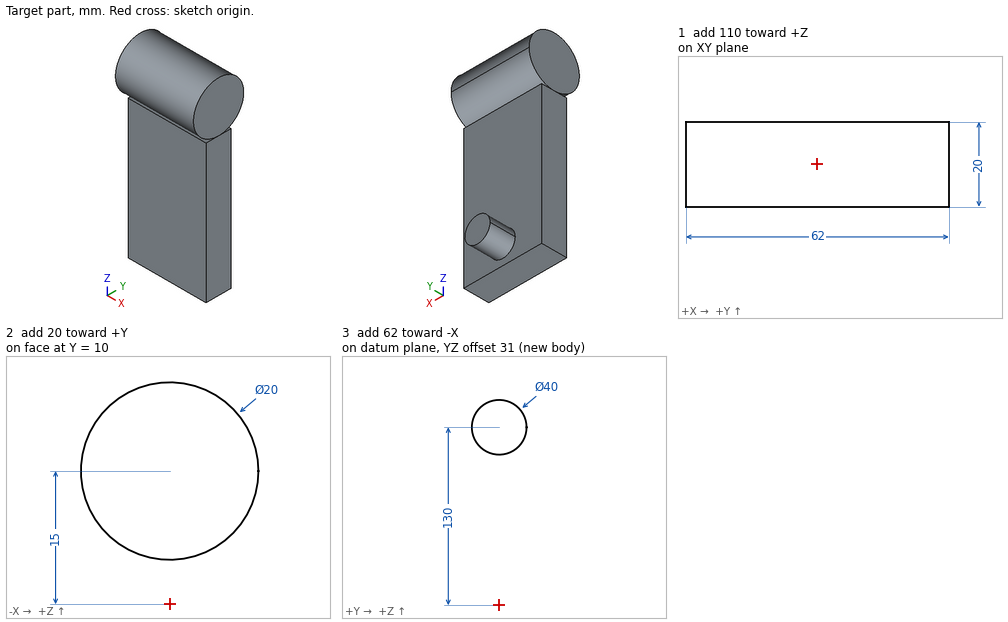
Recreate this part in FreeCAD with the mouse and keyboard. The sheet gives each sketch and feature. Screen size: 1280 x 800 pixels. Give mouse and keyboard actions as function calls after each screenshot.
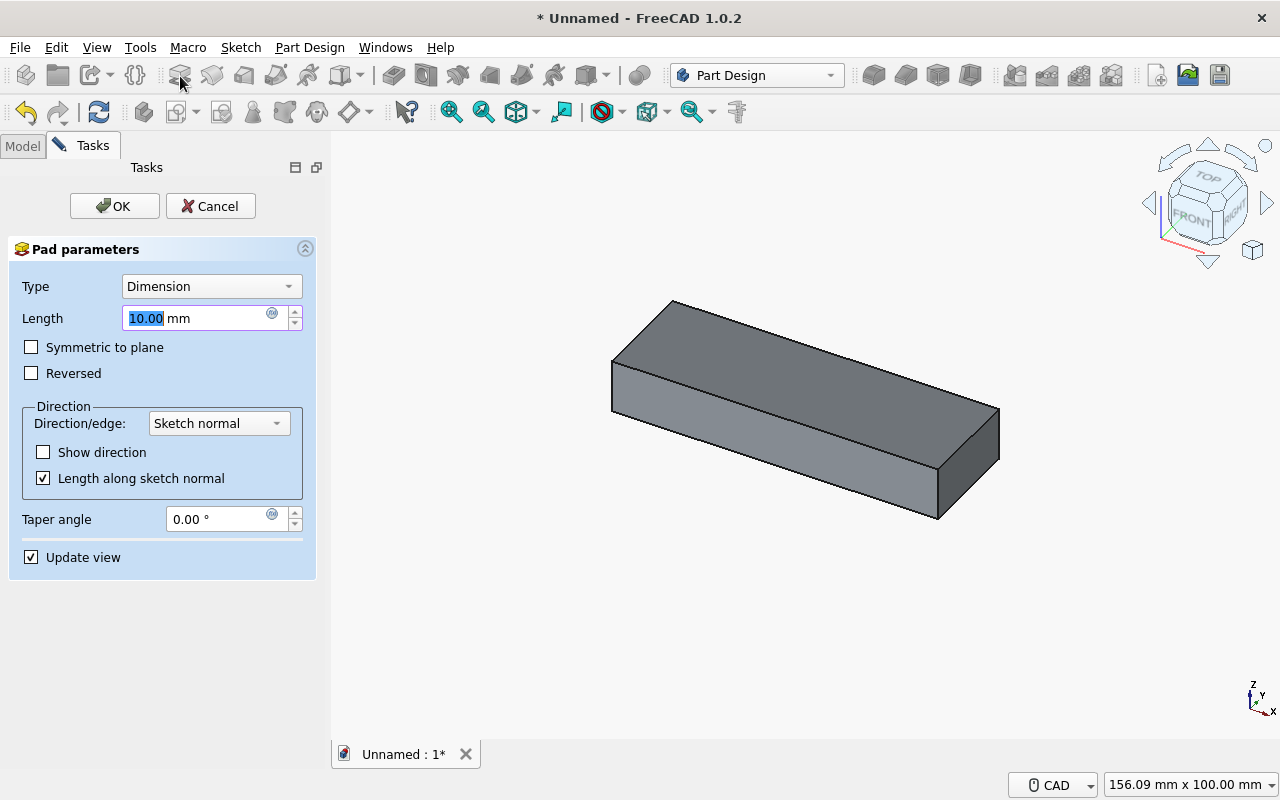
text(110)
key(Tab)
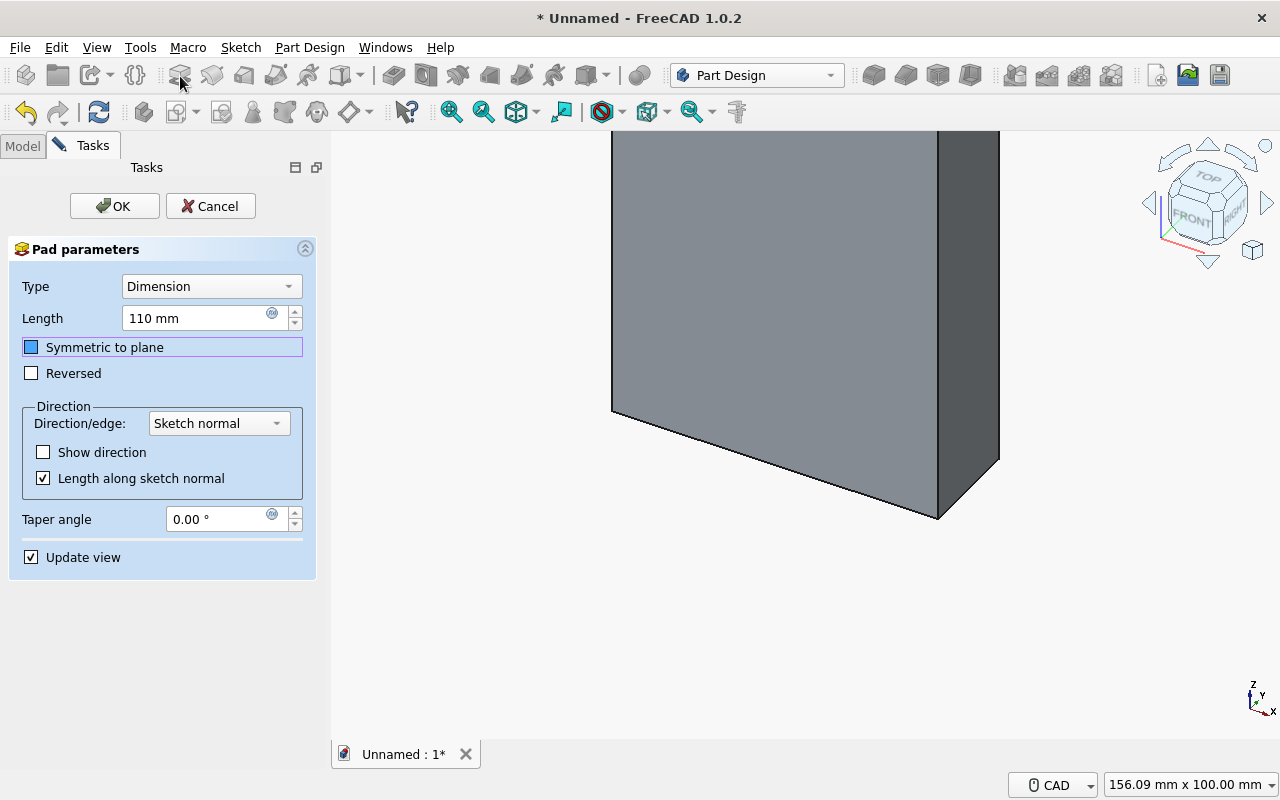
click(115, 206)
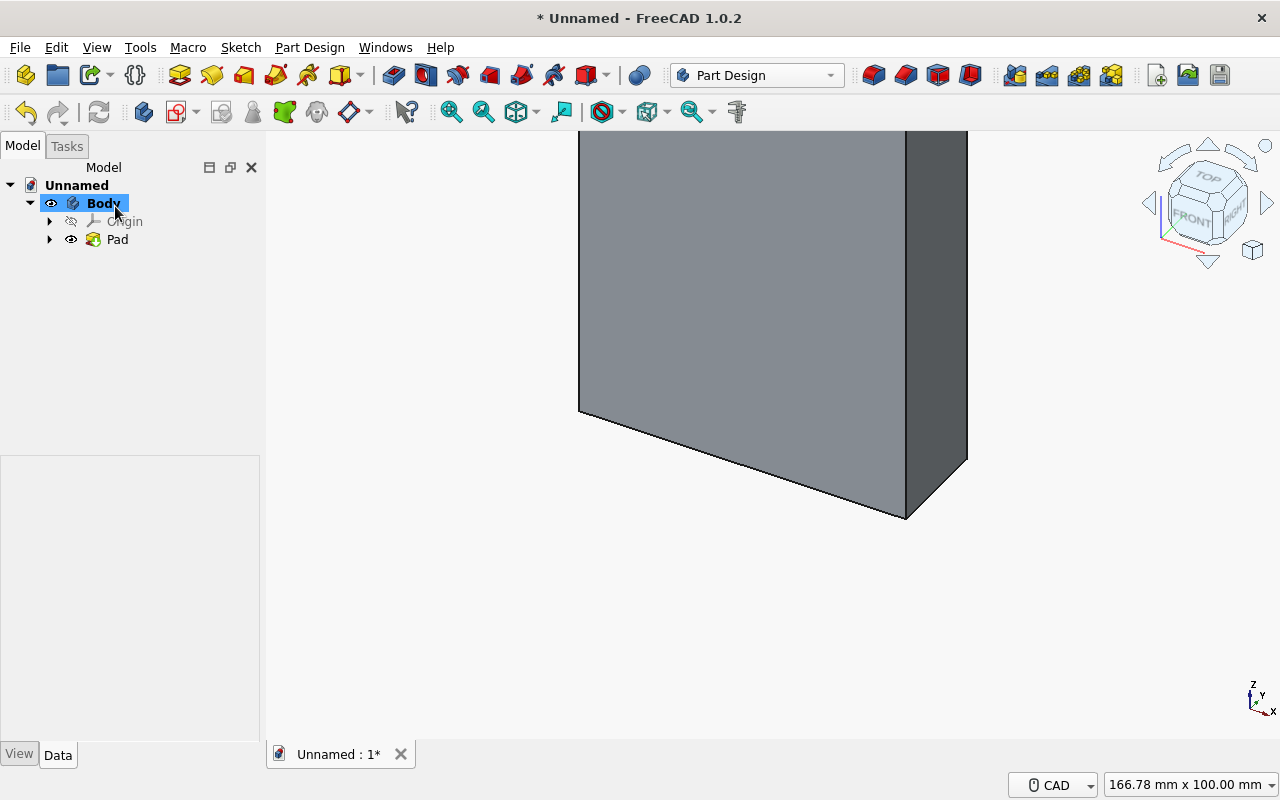
click(452, 112)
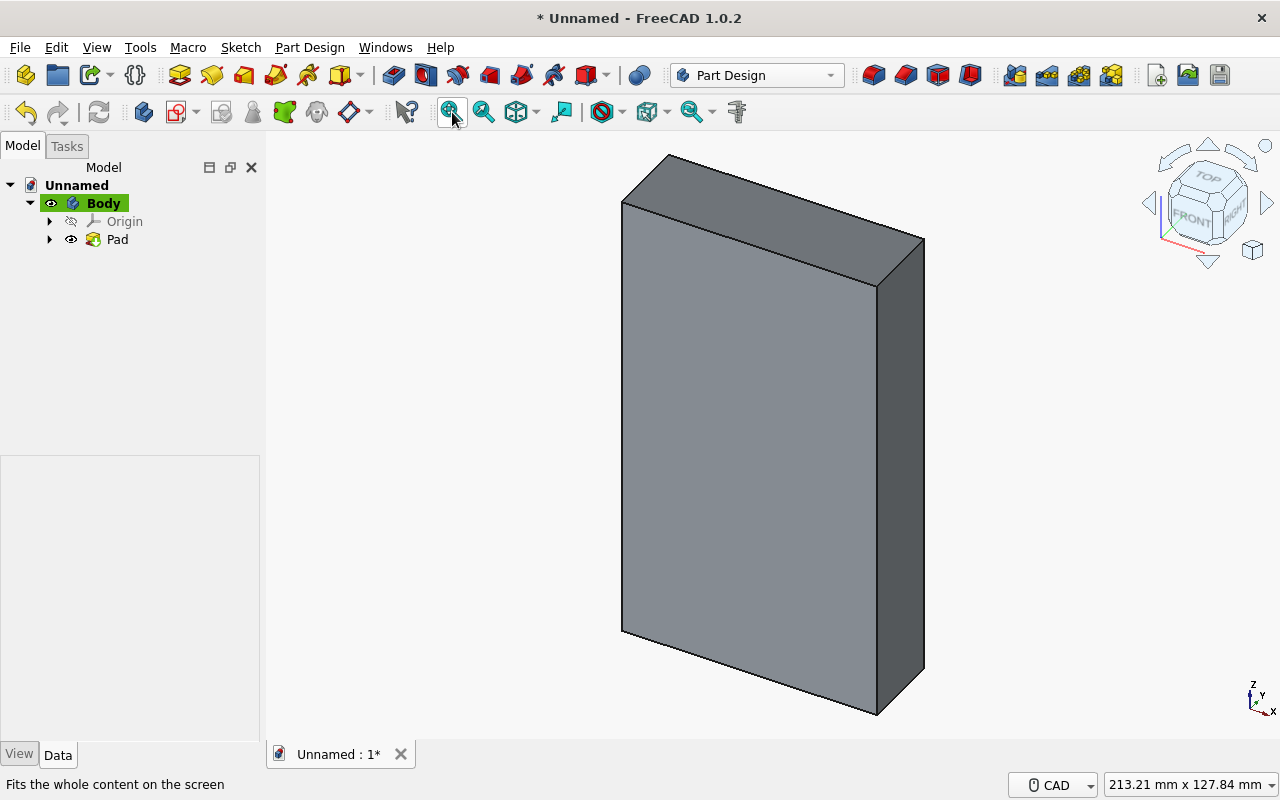
key(4)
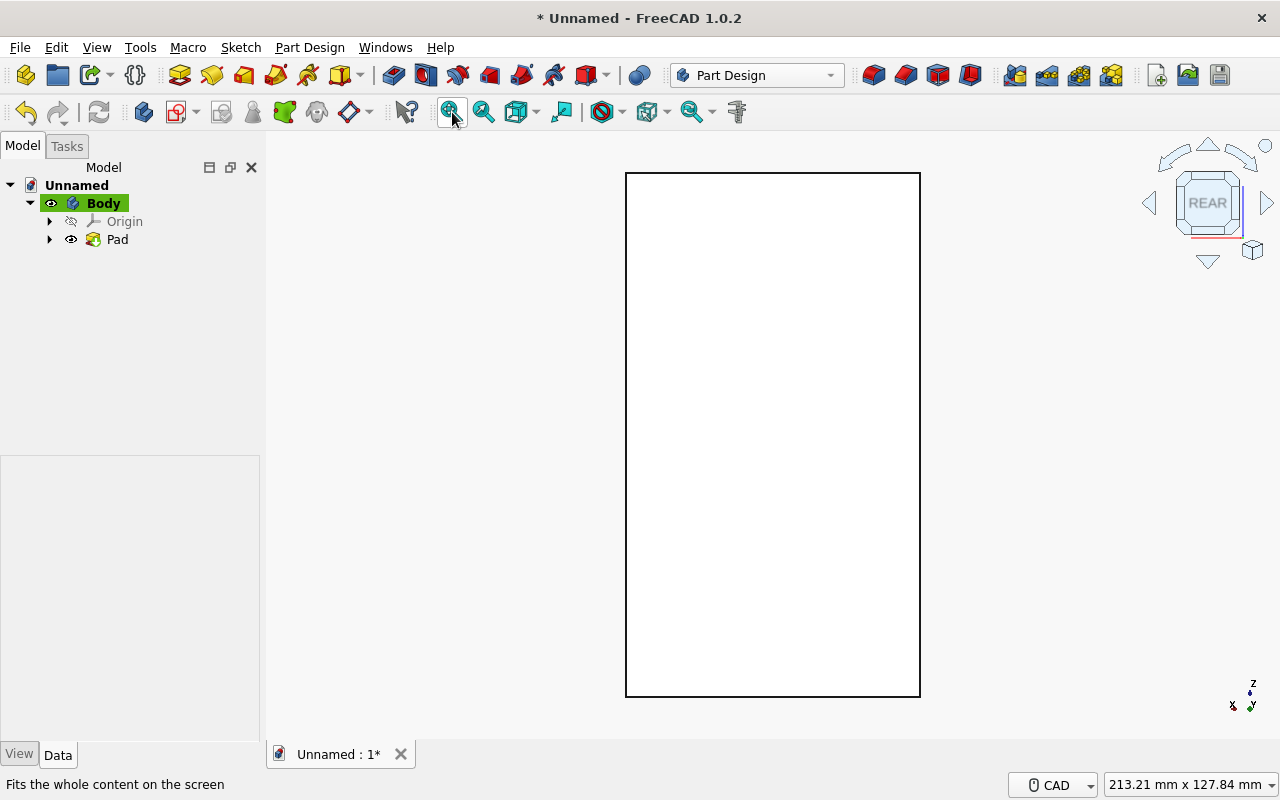
click(773, 359)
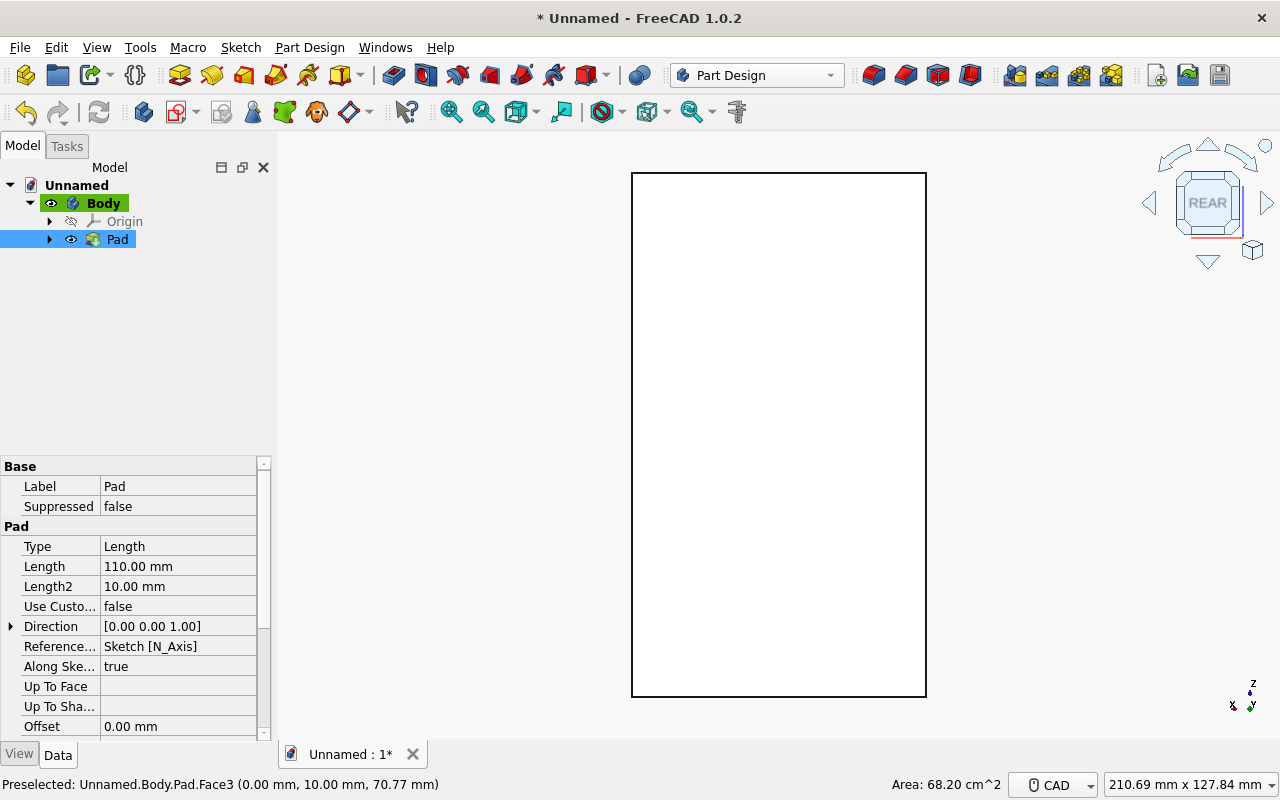
click(176, 112)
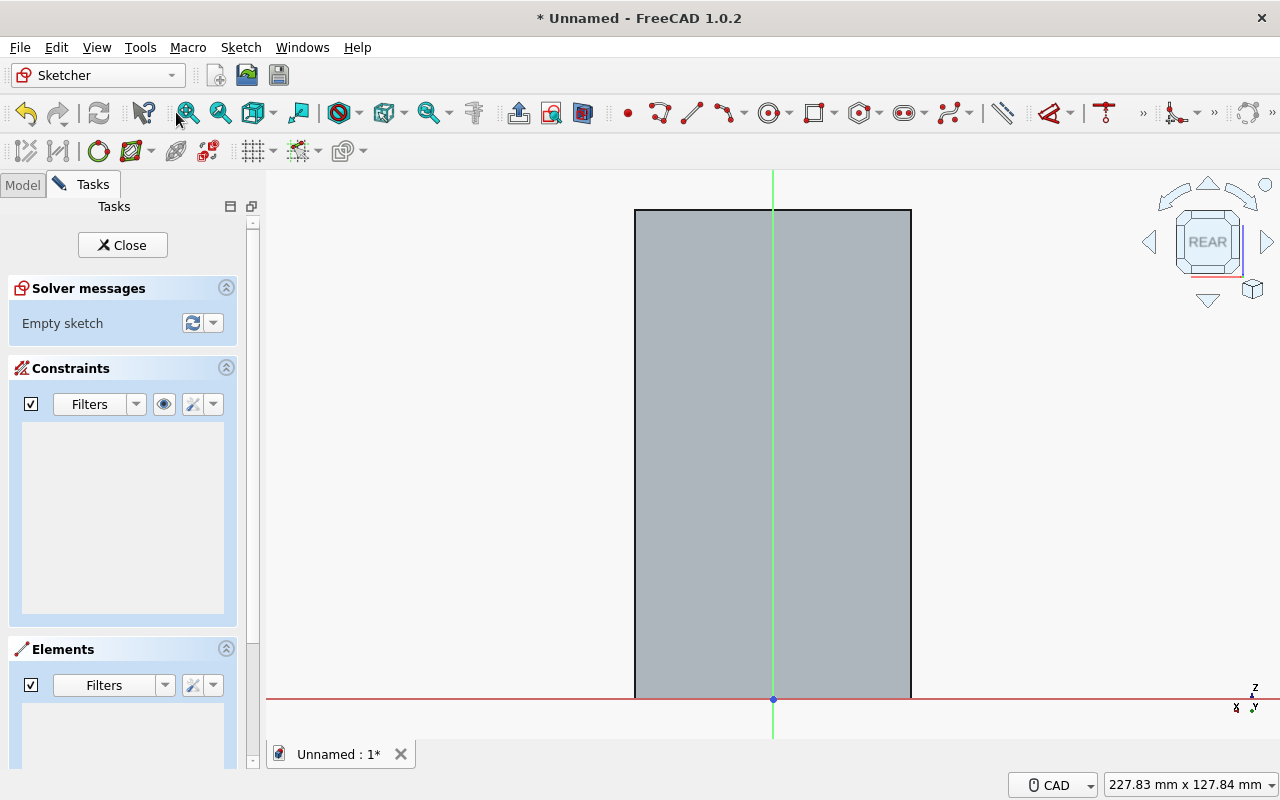
scroll(803, 711, up, 6)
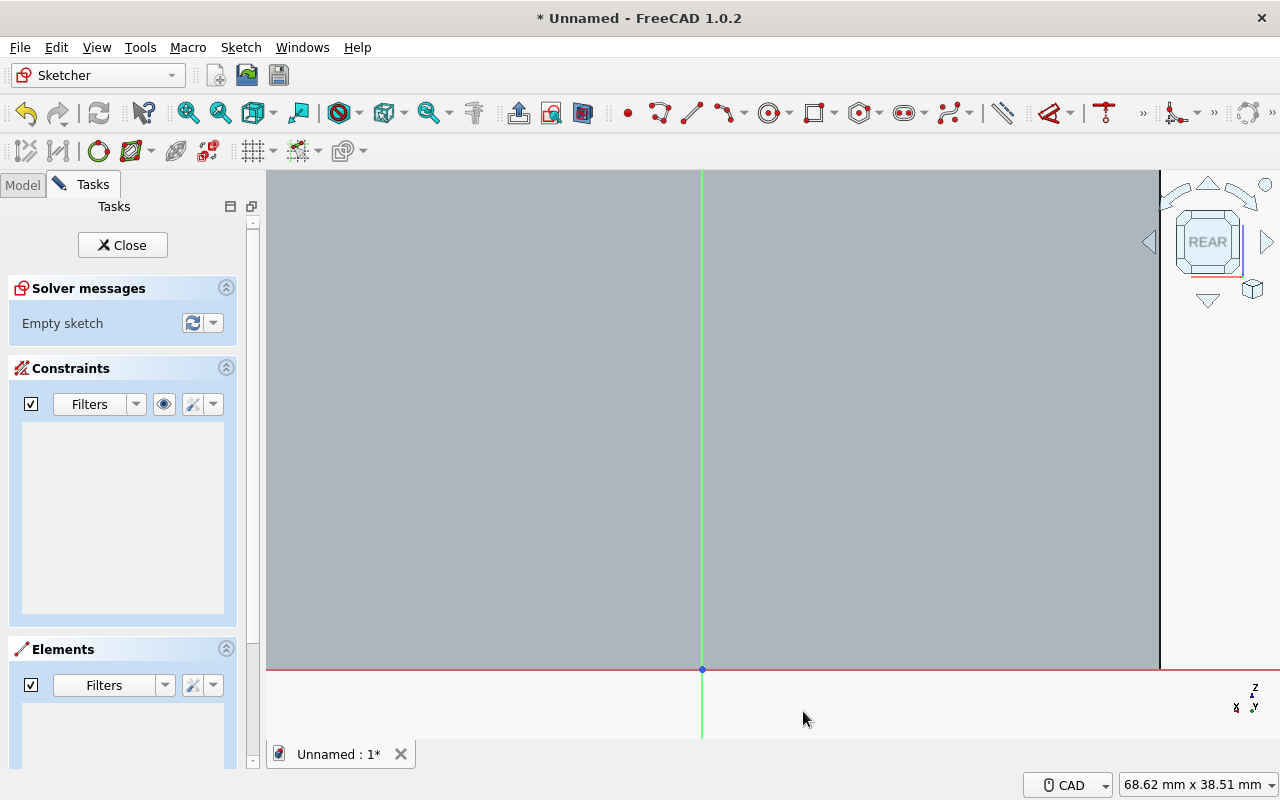
key(g)
key(c)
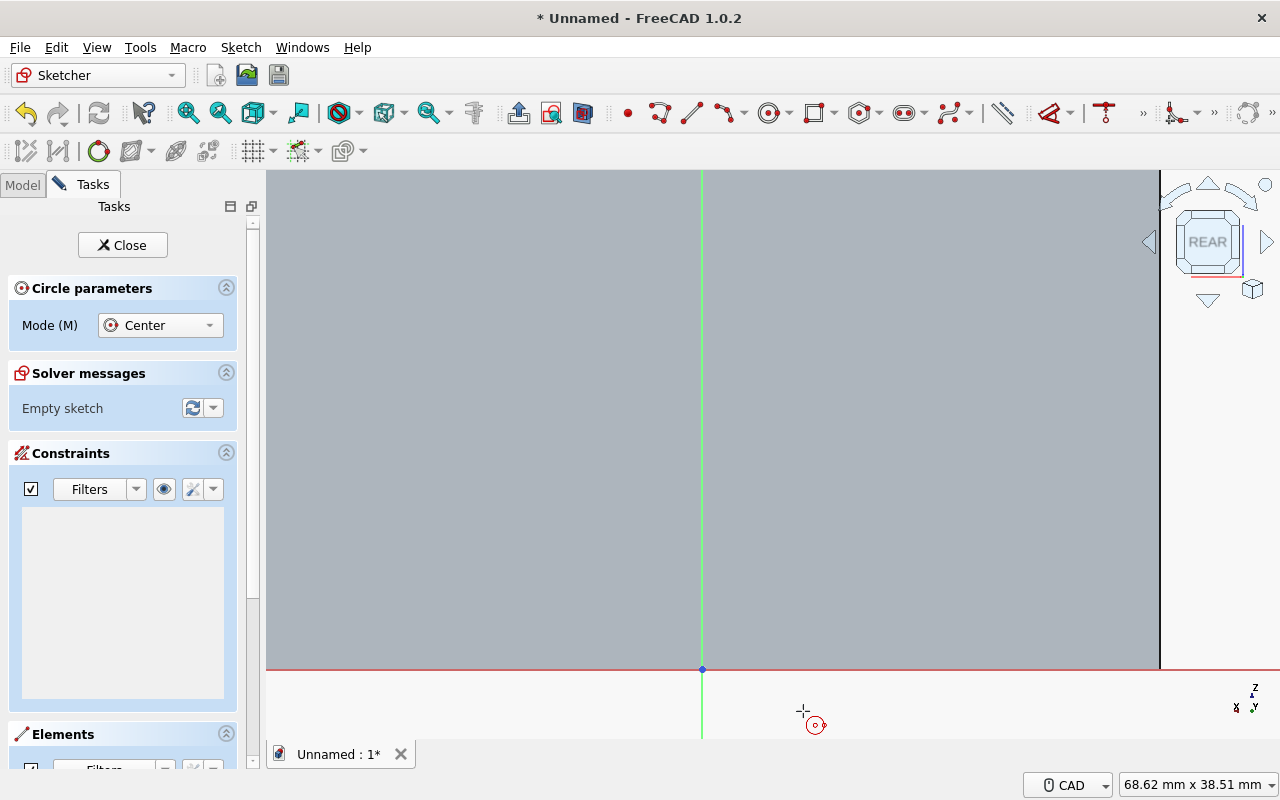
click(702, 448)
move(807, 344)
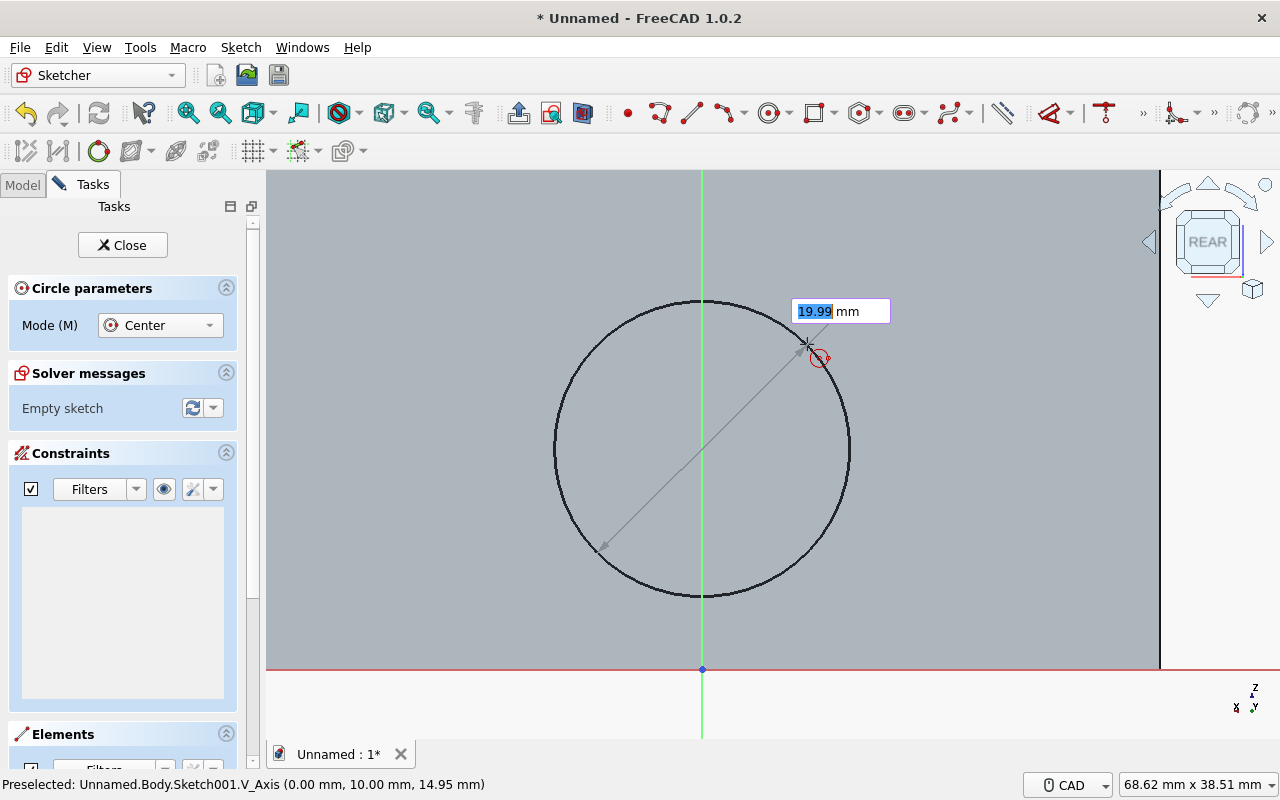
text(20)
key(Return)
key(Escape)